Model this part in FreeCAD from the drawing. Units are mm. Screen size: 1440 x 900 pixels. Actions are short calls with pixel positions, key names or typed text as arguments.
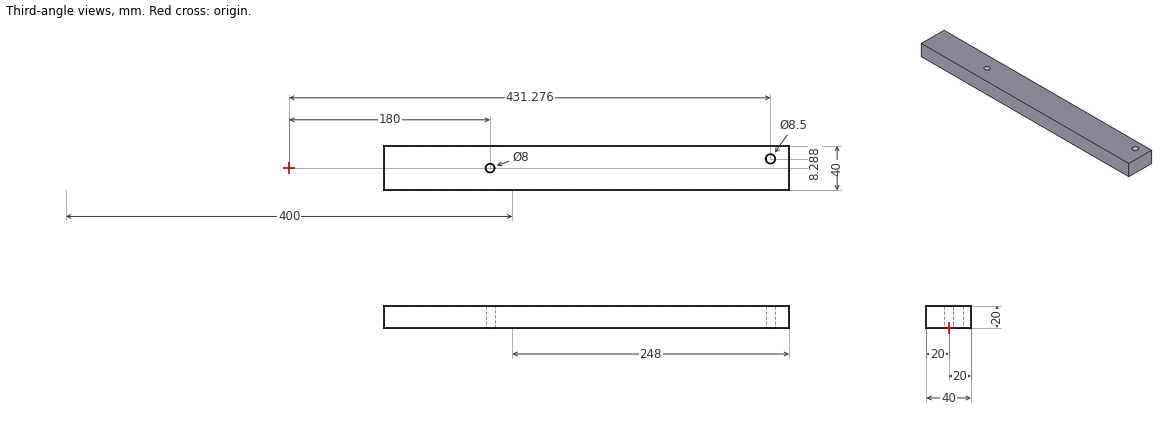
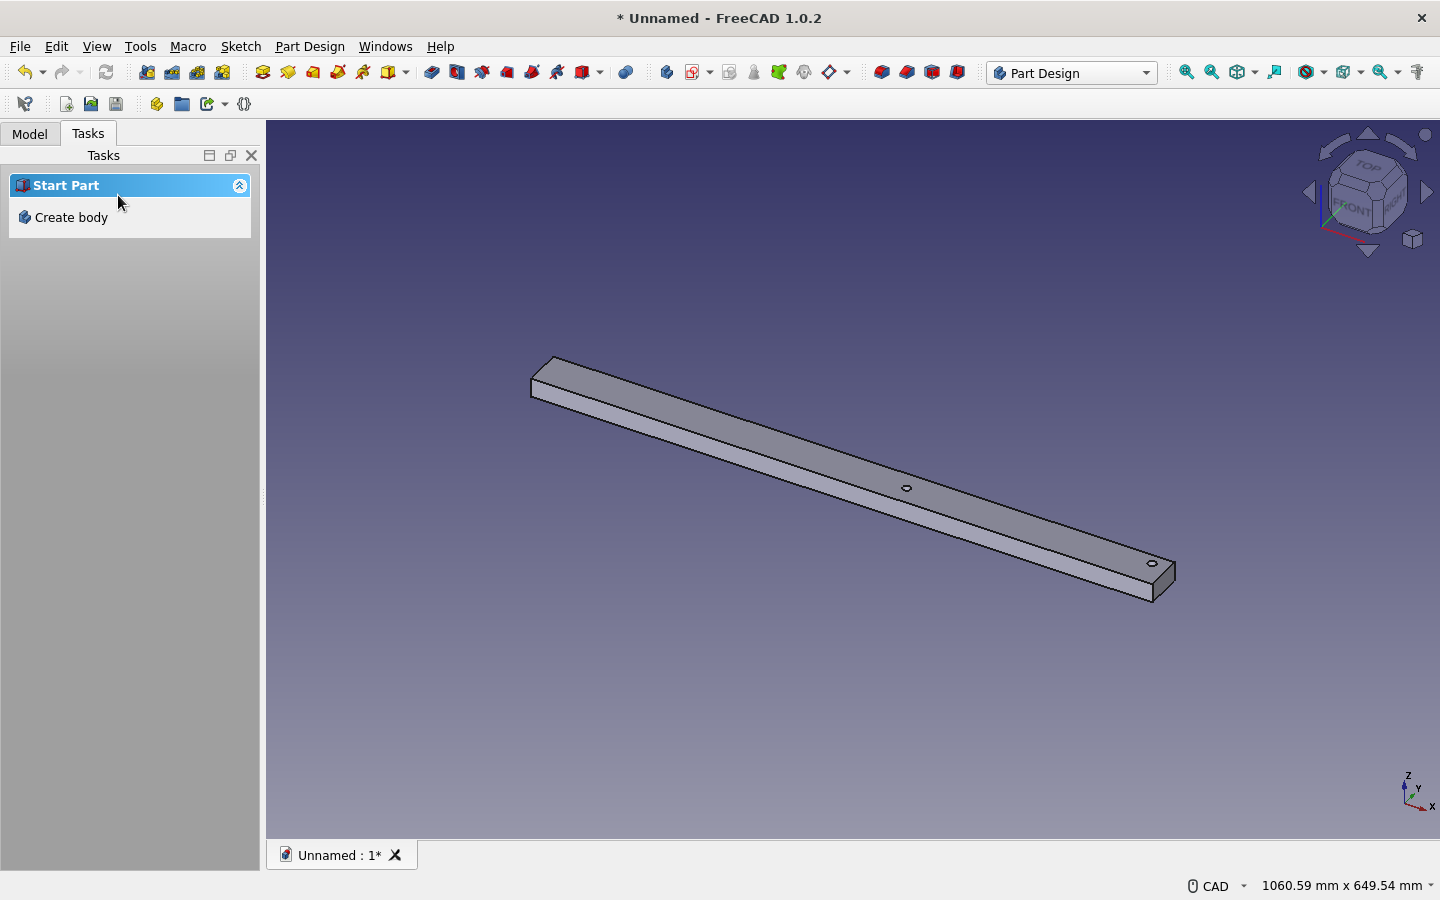
key(6)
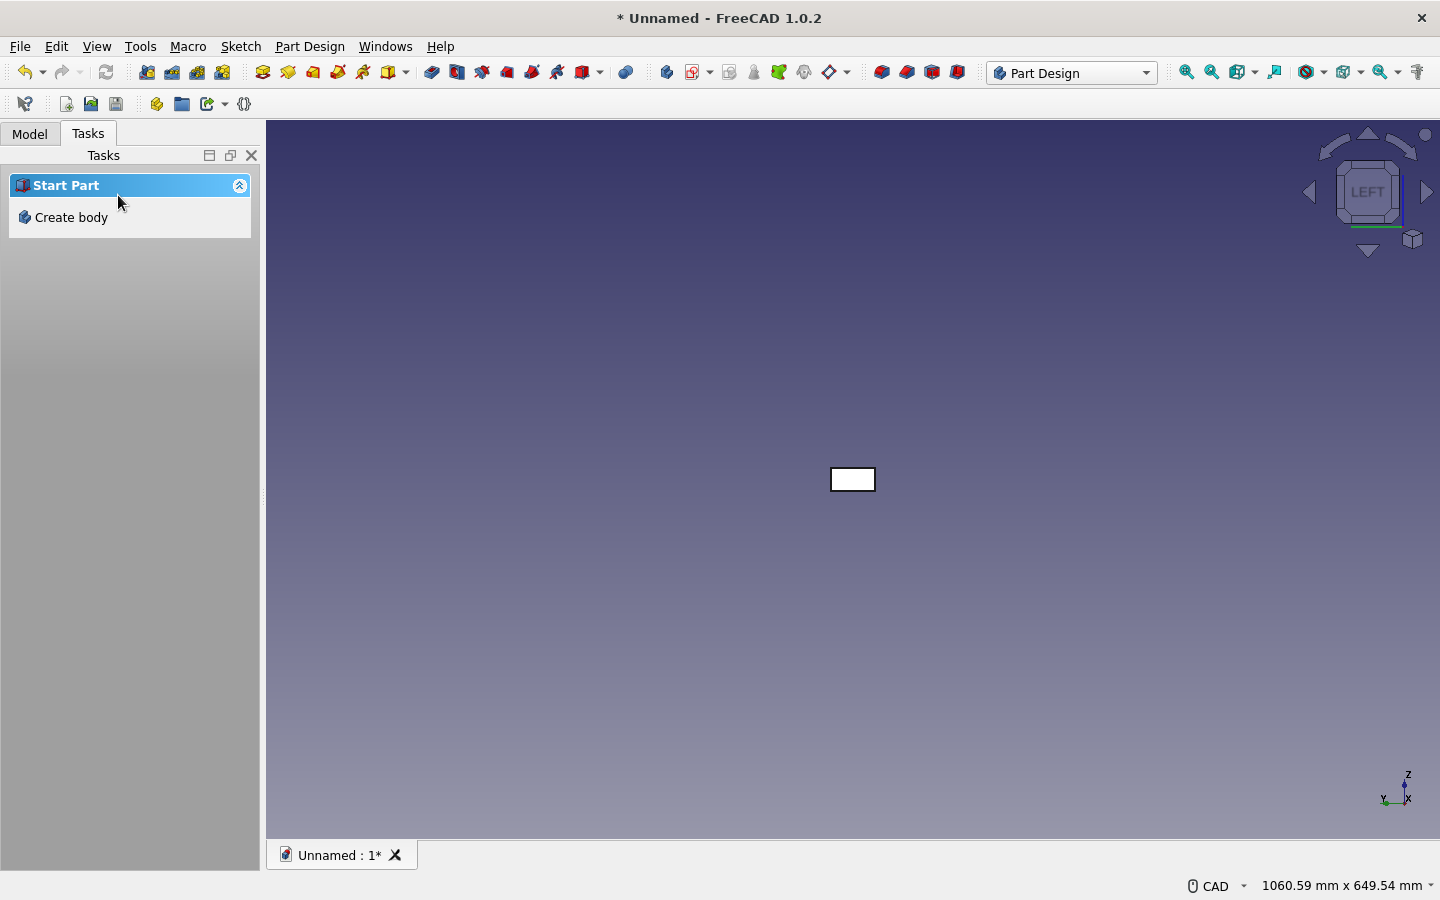
click(1187, 72)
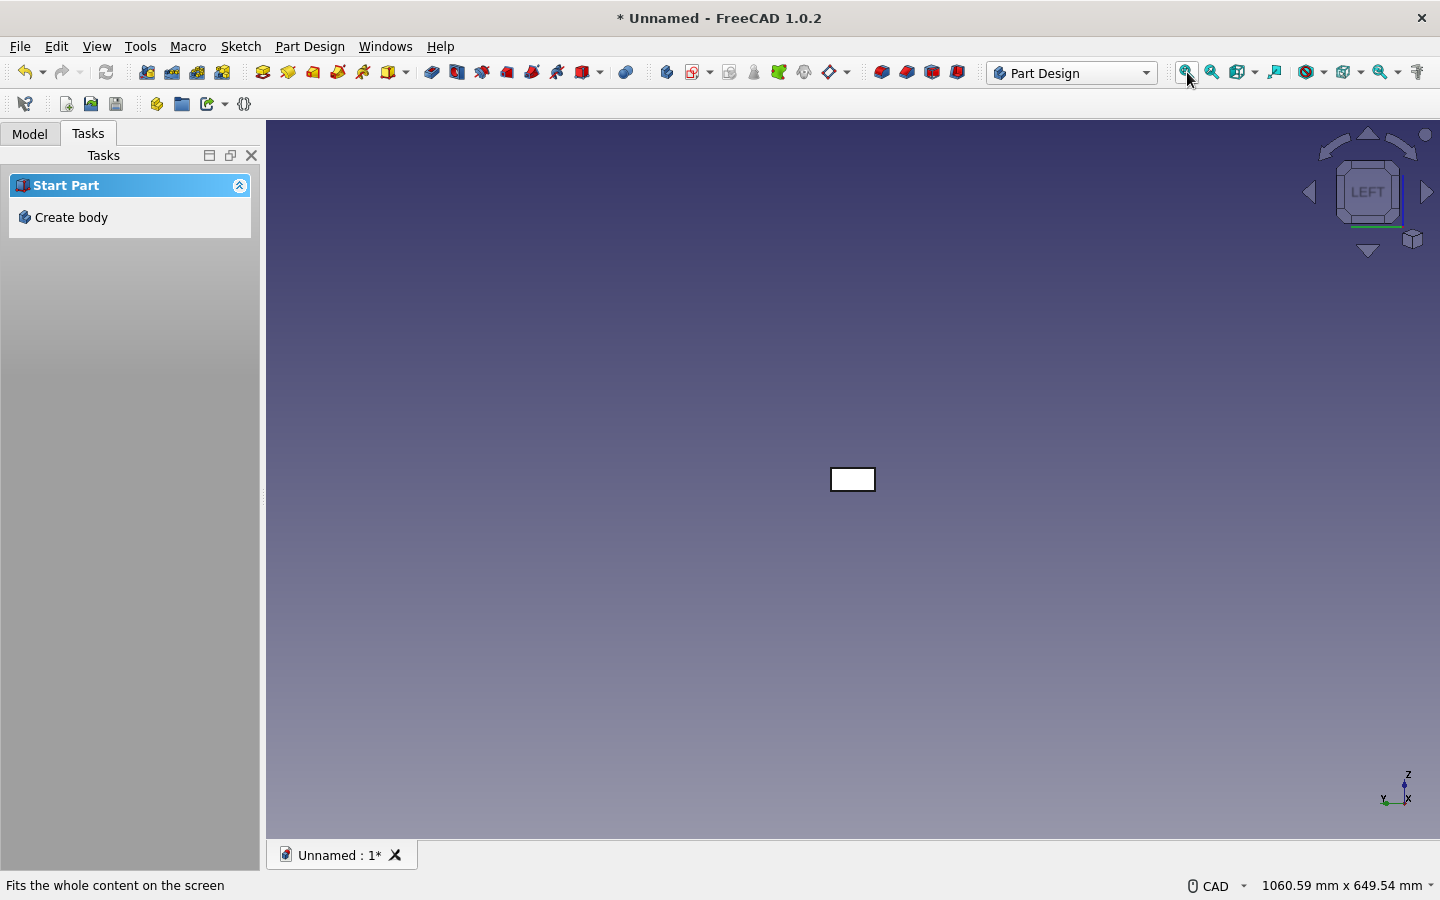
click(847, 478)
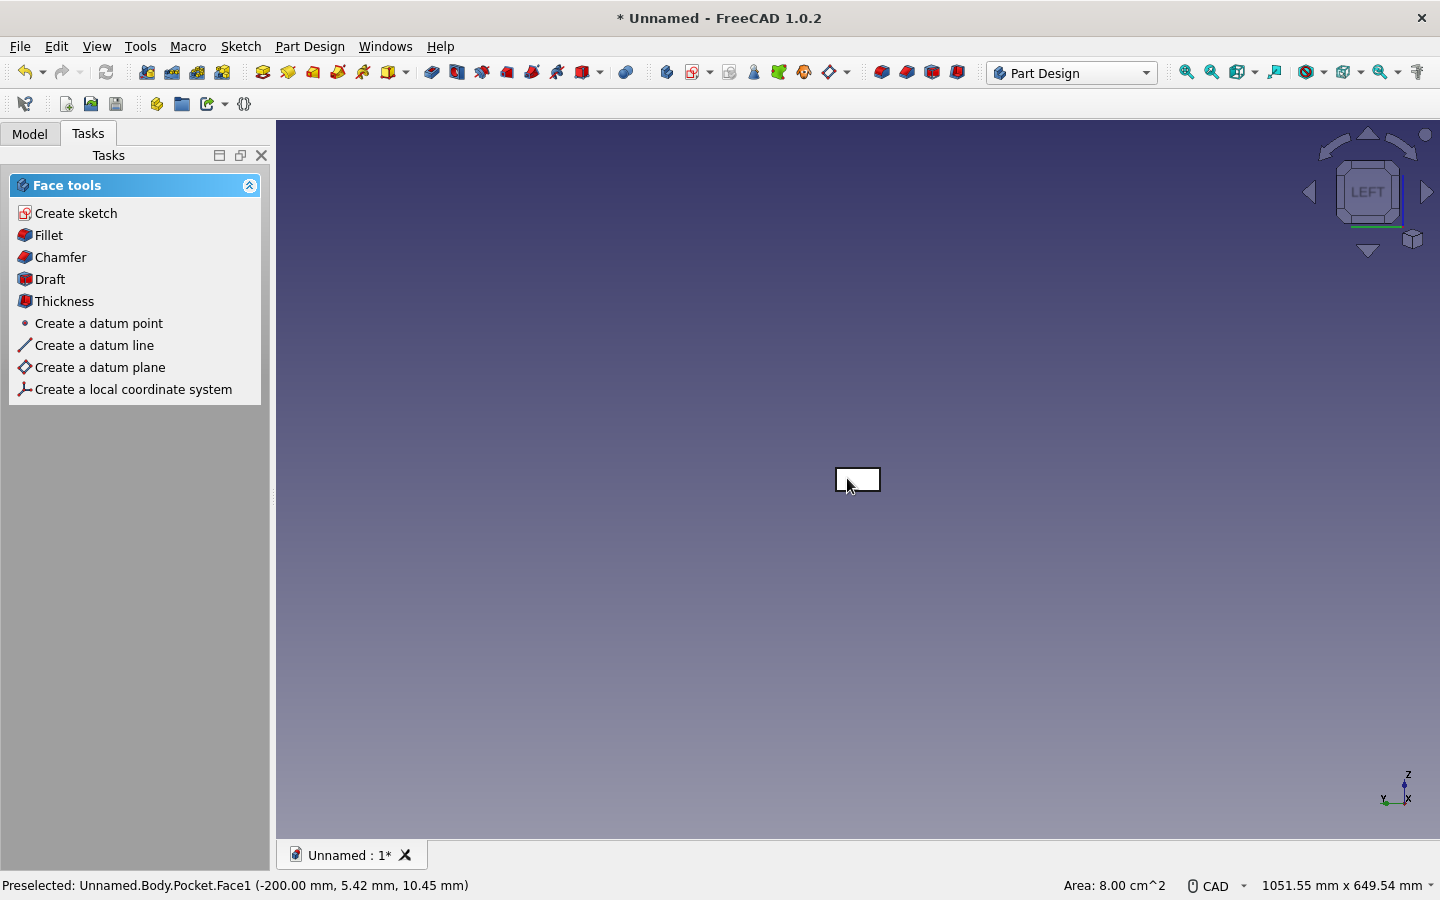
click(692, 72)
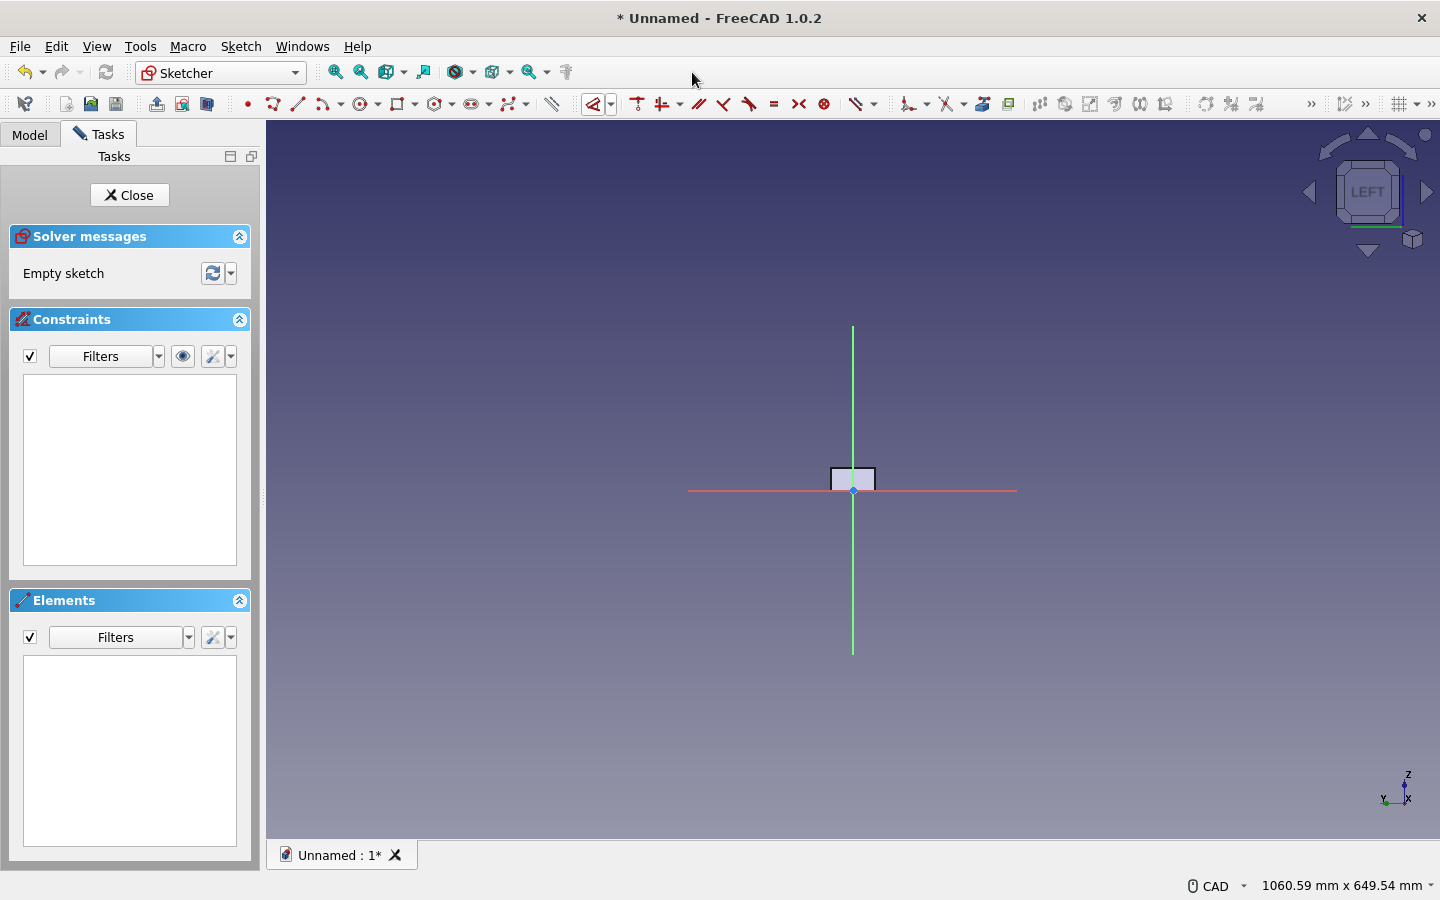
scroll(857, 480, up, 14)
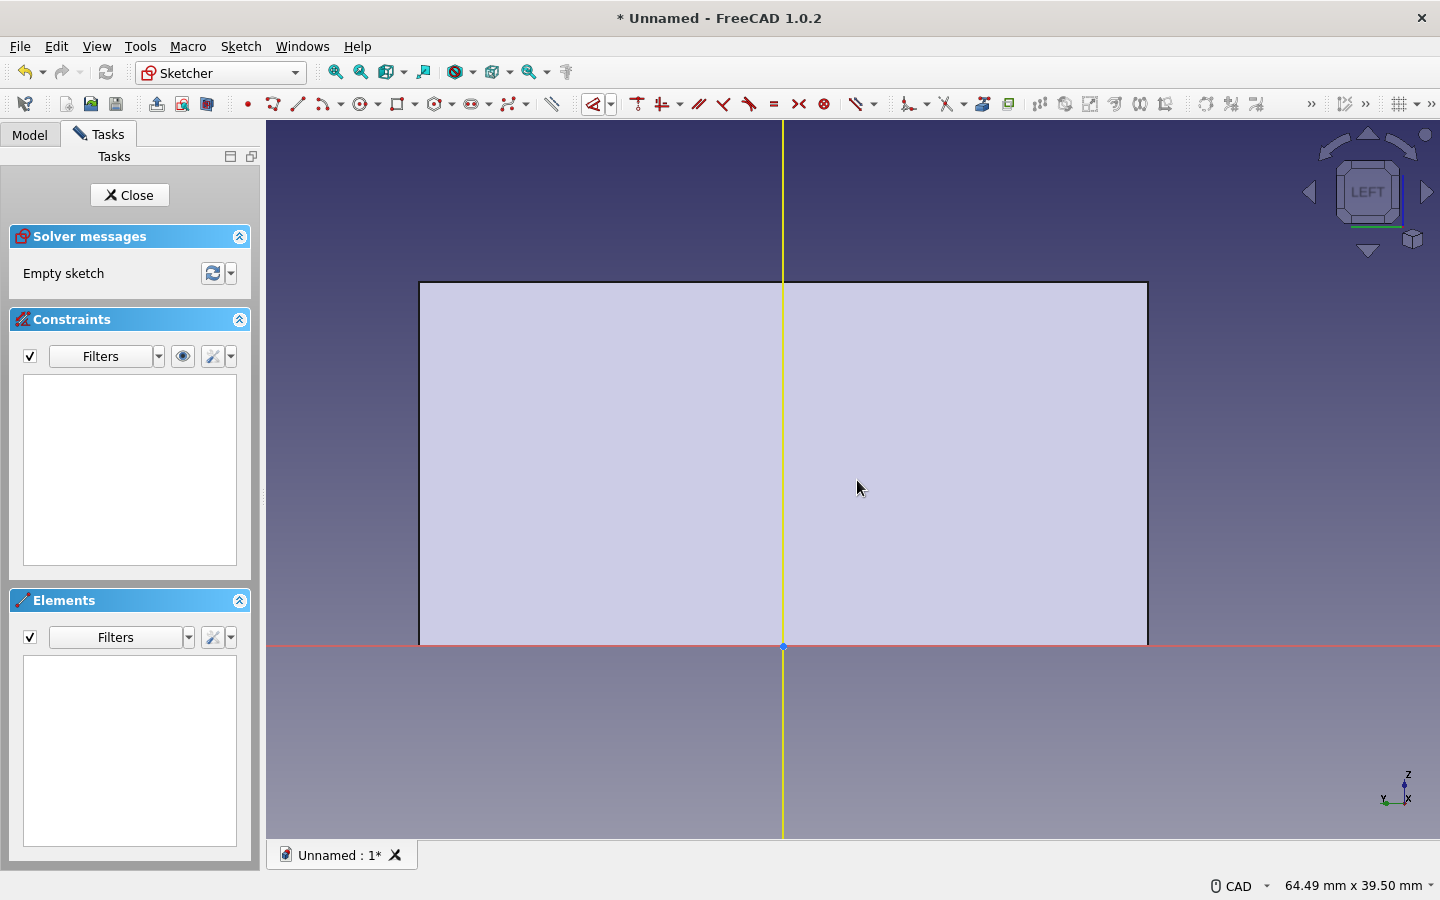
click(396, 104)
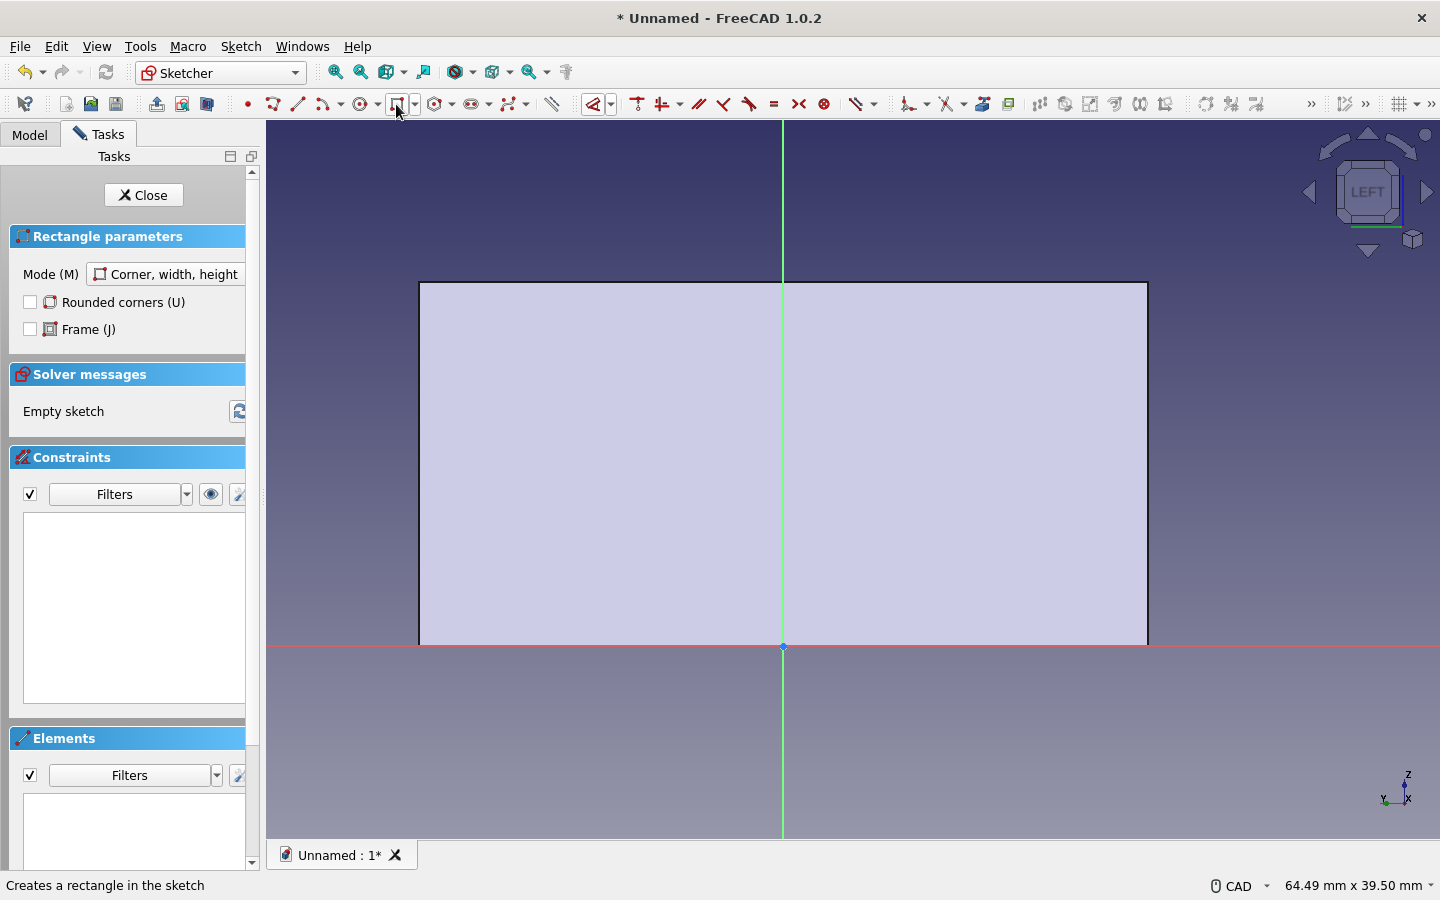
click(419, 282)
click(1148, 646)
key(Escape)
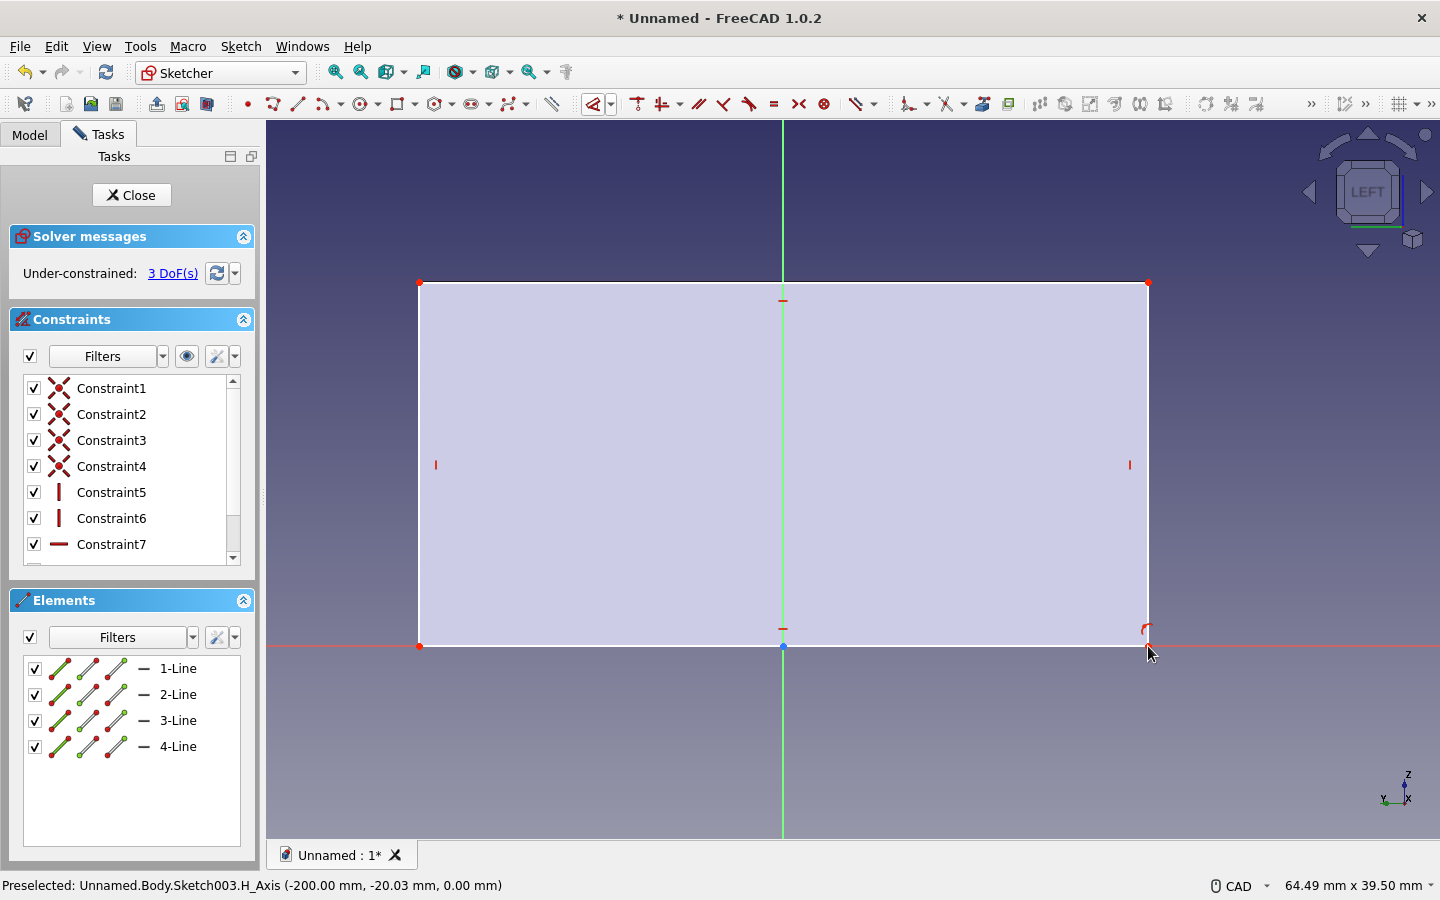
click(419, 392)